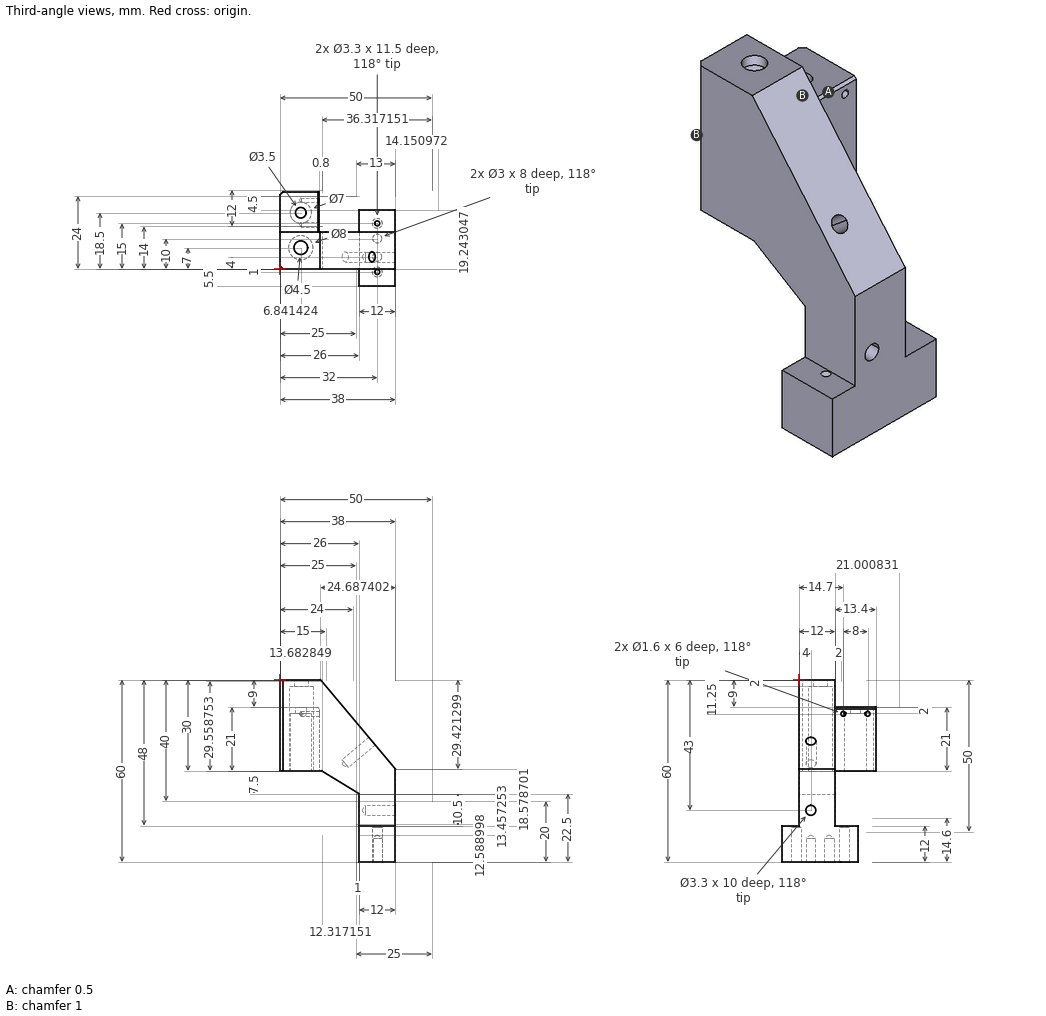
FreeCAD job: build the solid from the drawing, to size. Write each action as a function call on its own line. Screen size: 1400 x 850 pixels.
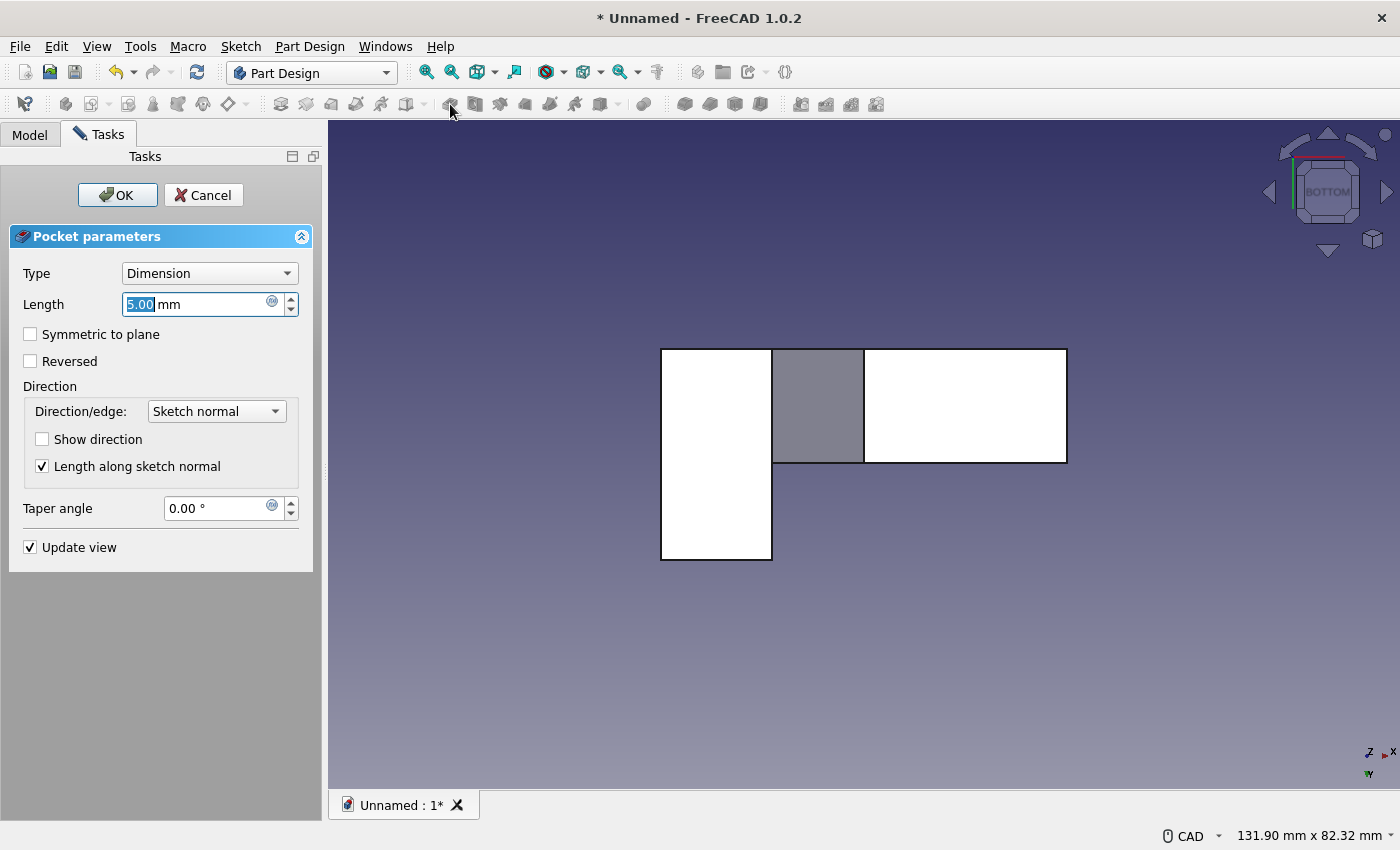
text(50)
key(Tab)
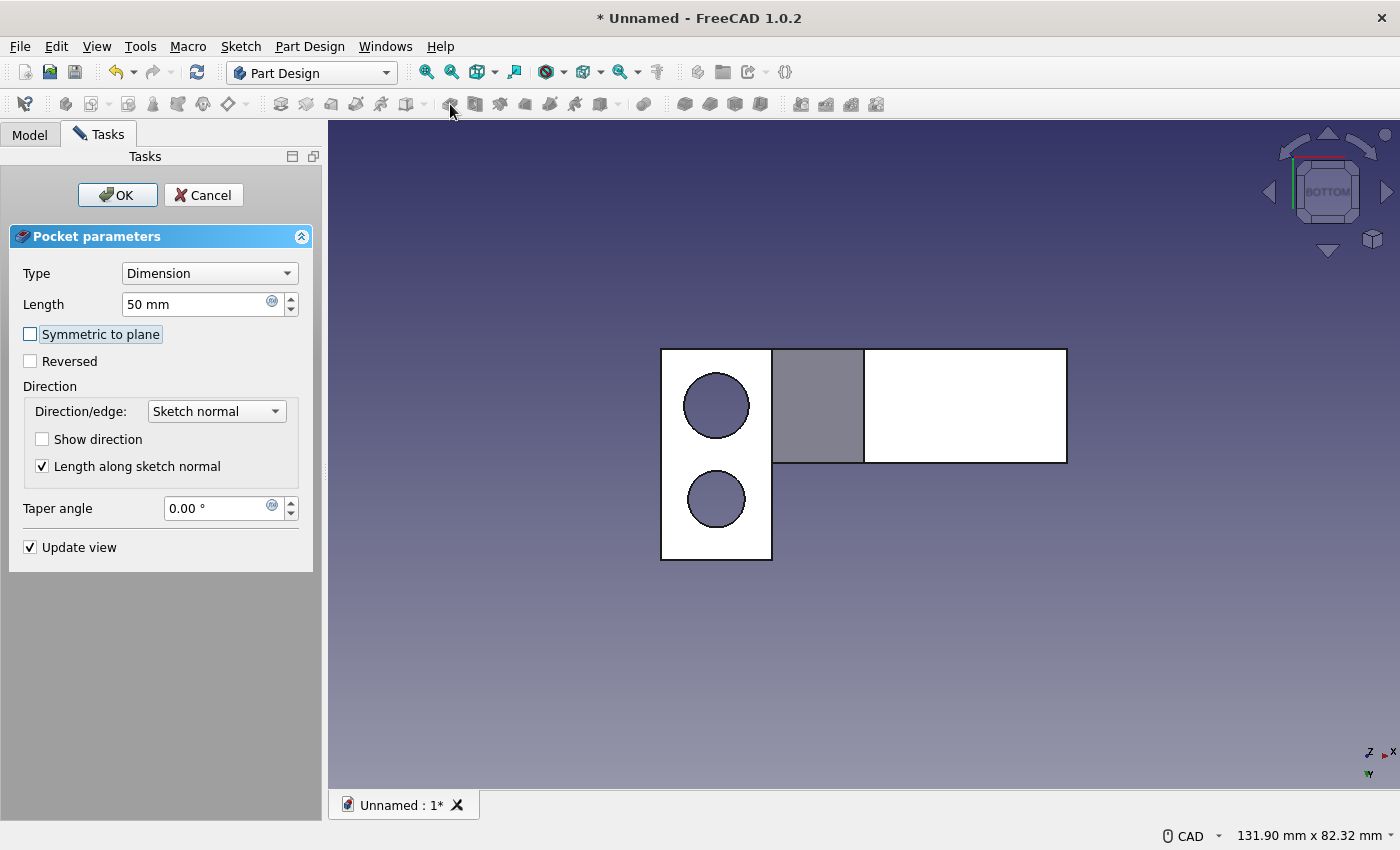
click(118, 195)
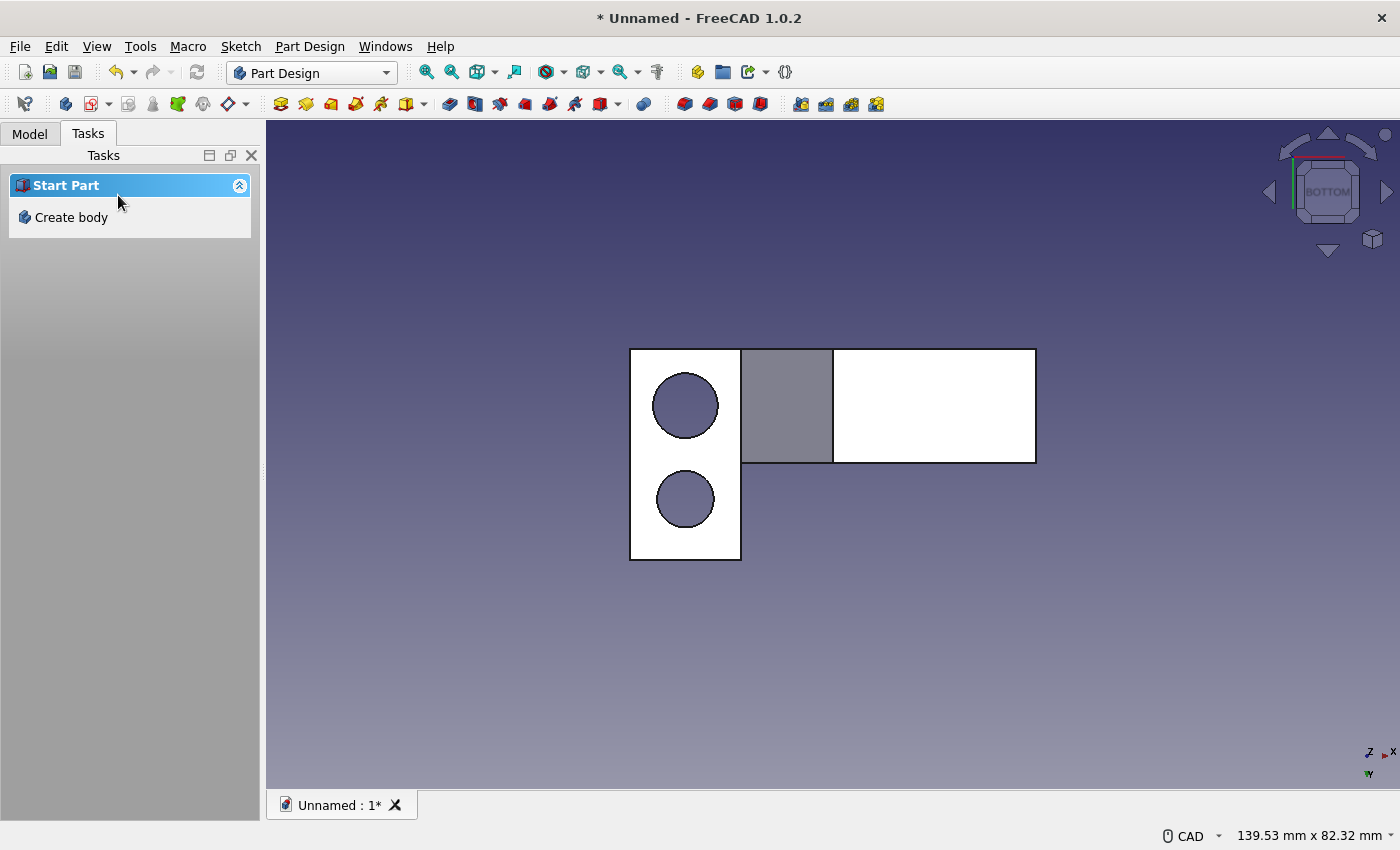
key(v)
key(f)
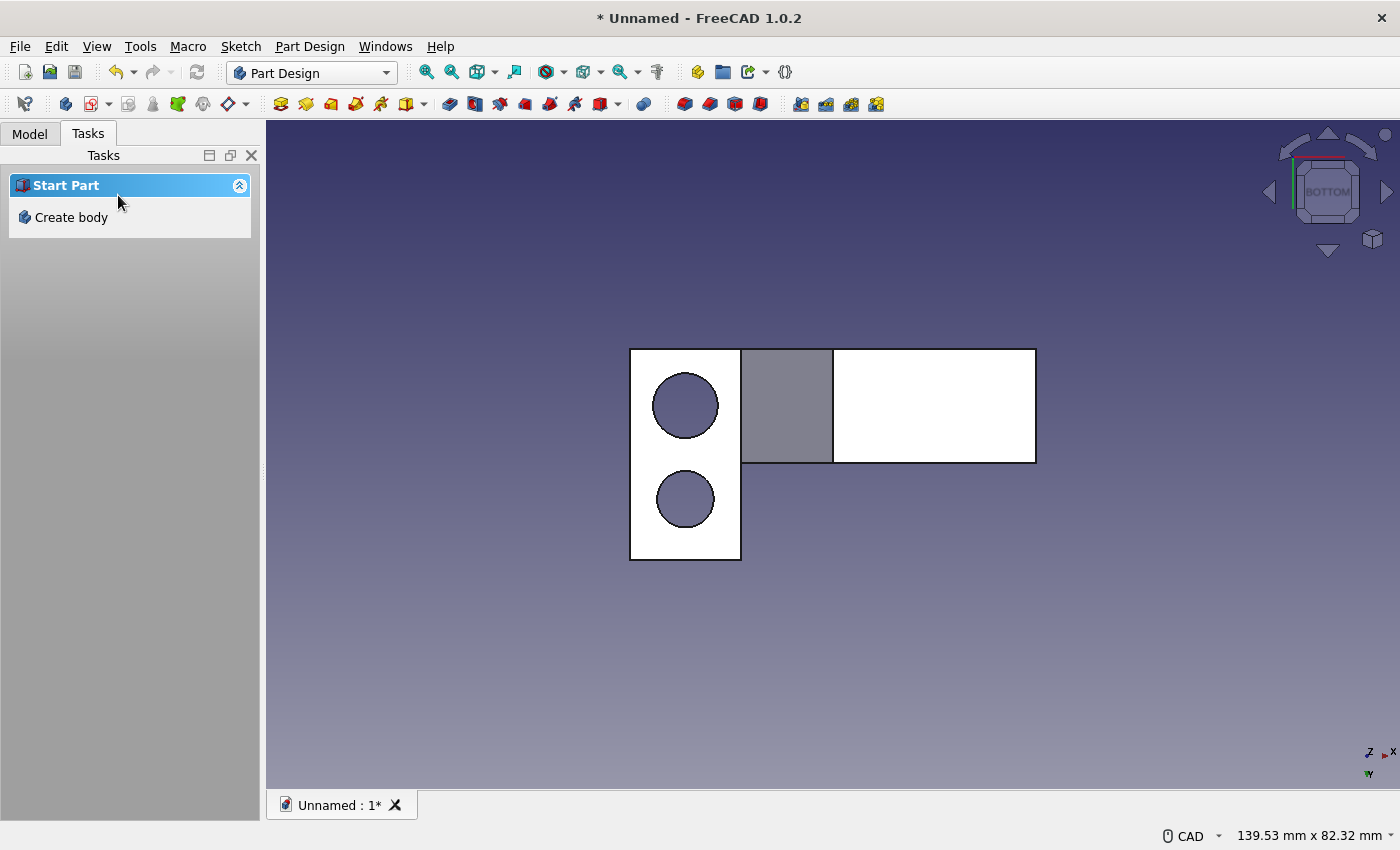
click(90, 104)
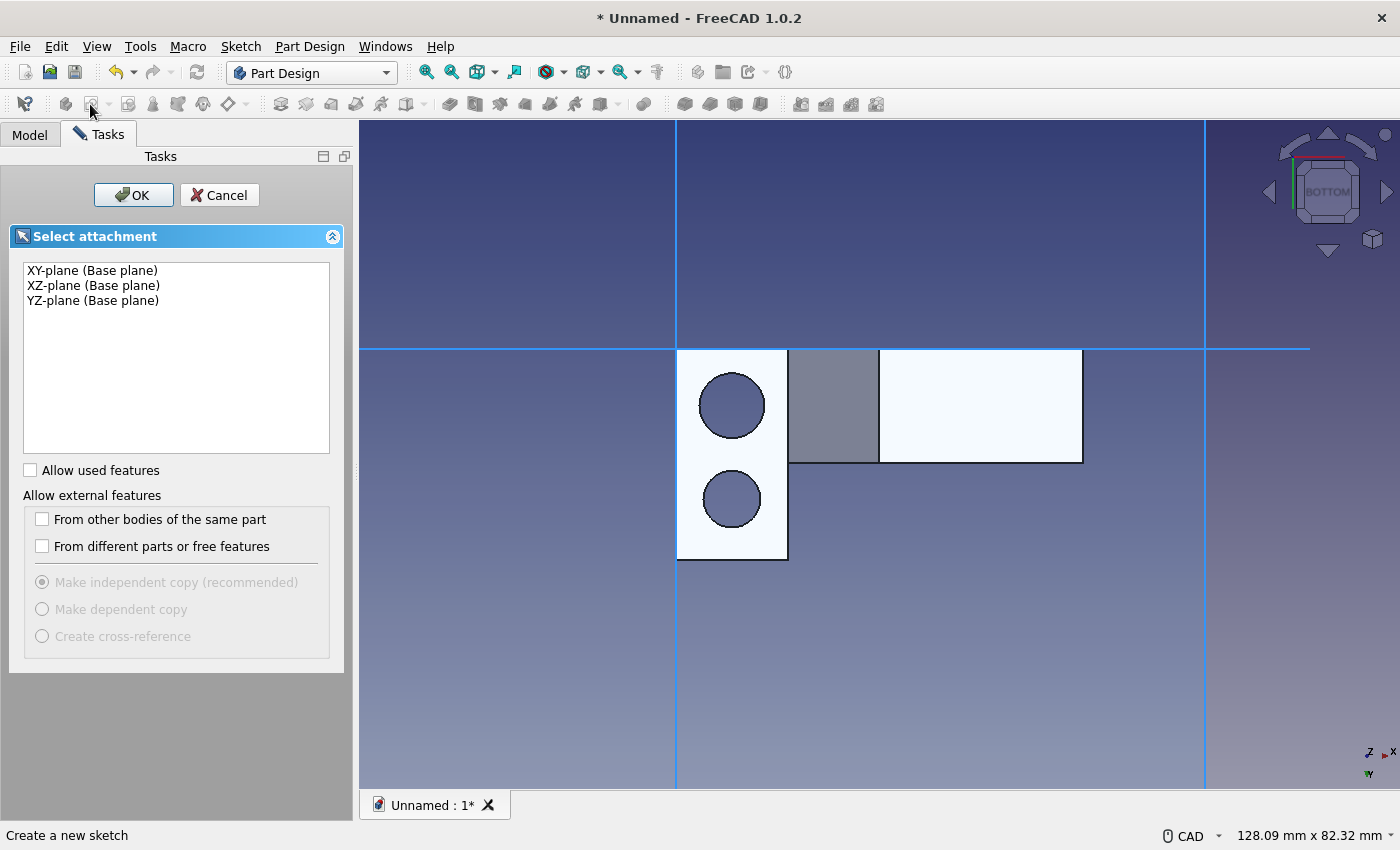
click(84, 270)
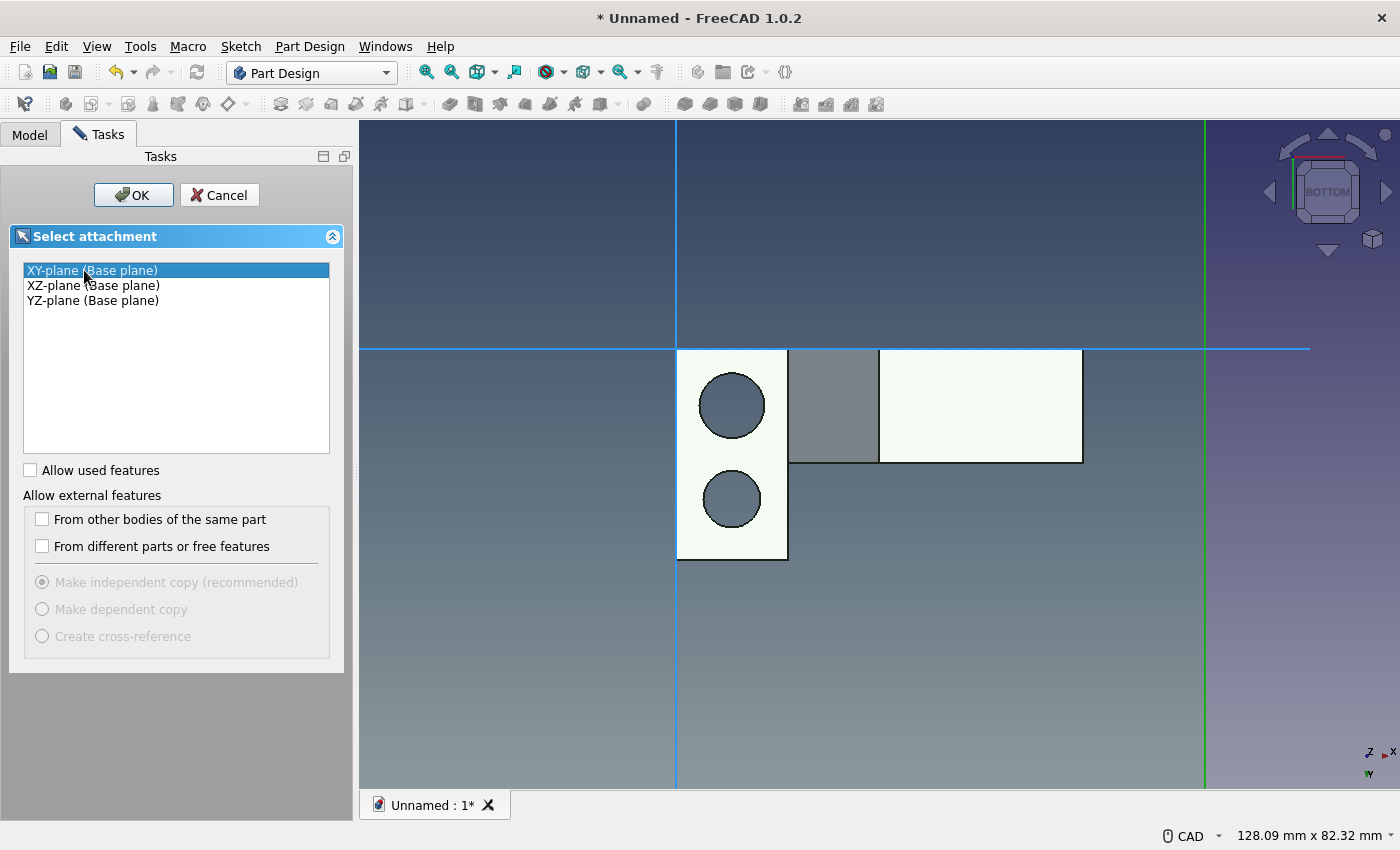
click(134, 195)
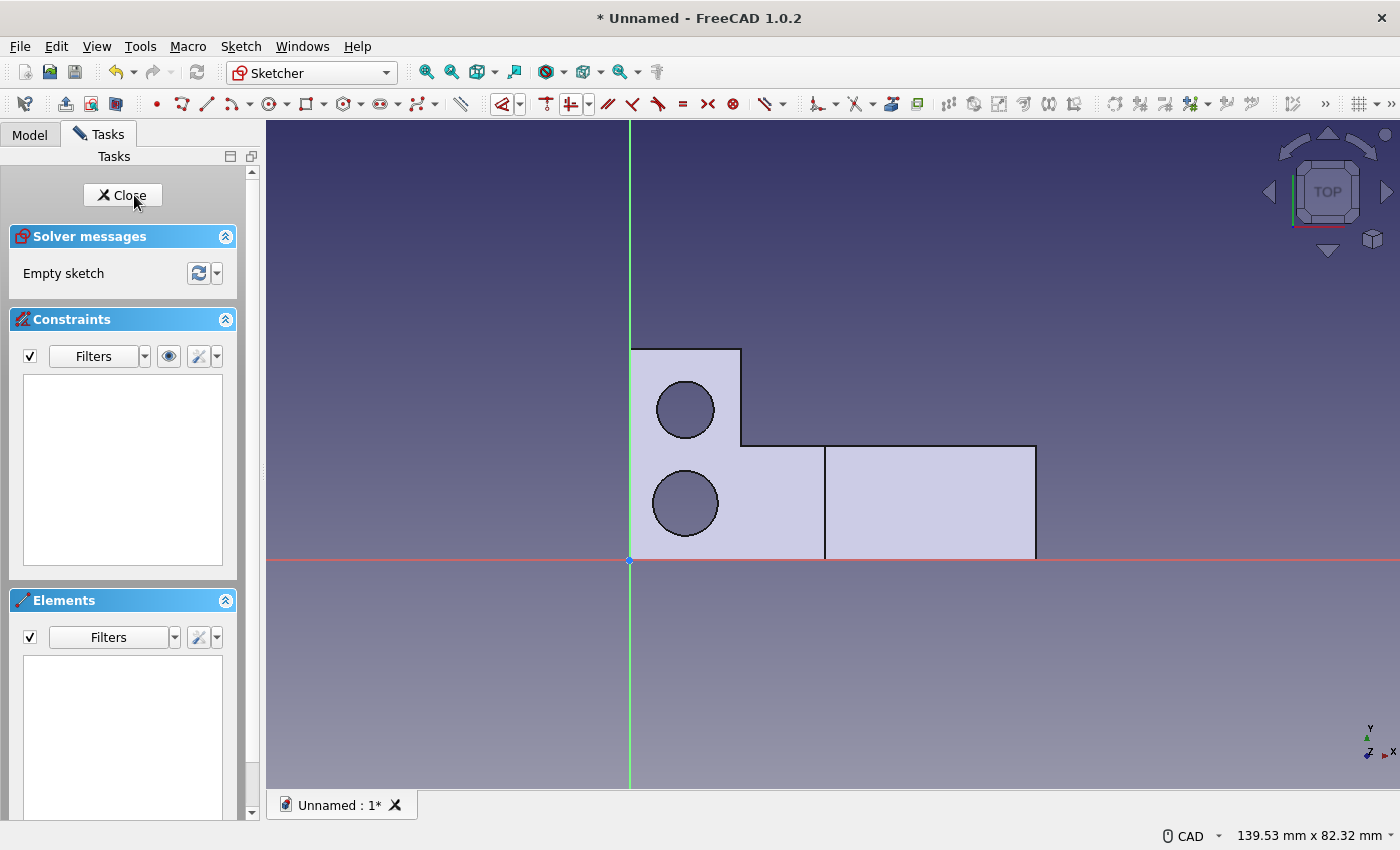
scroll(651, 531, up, 8)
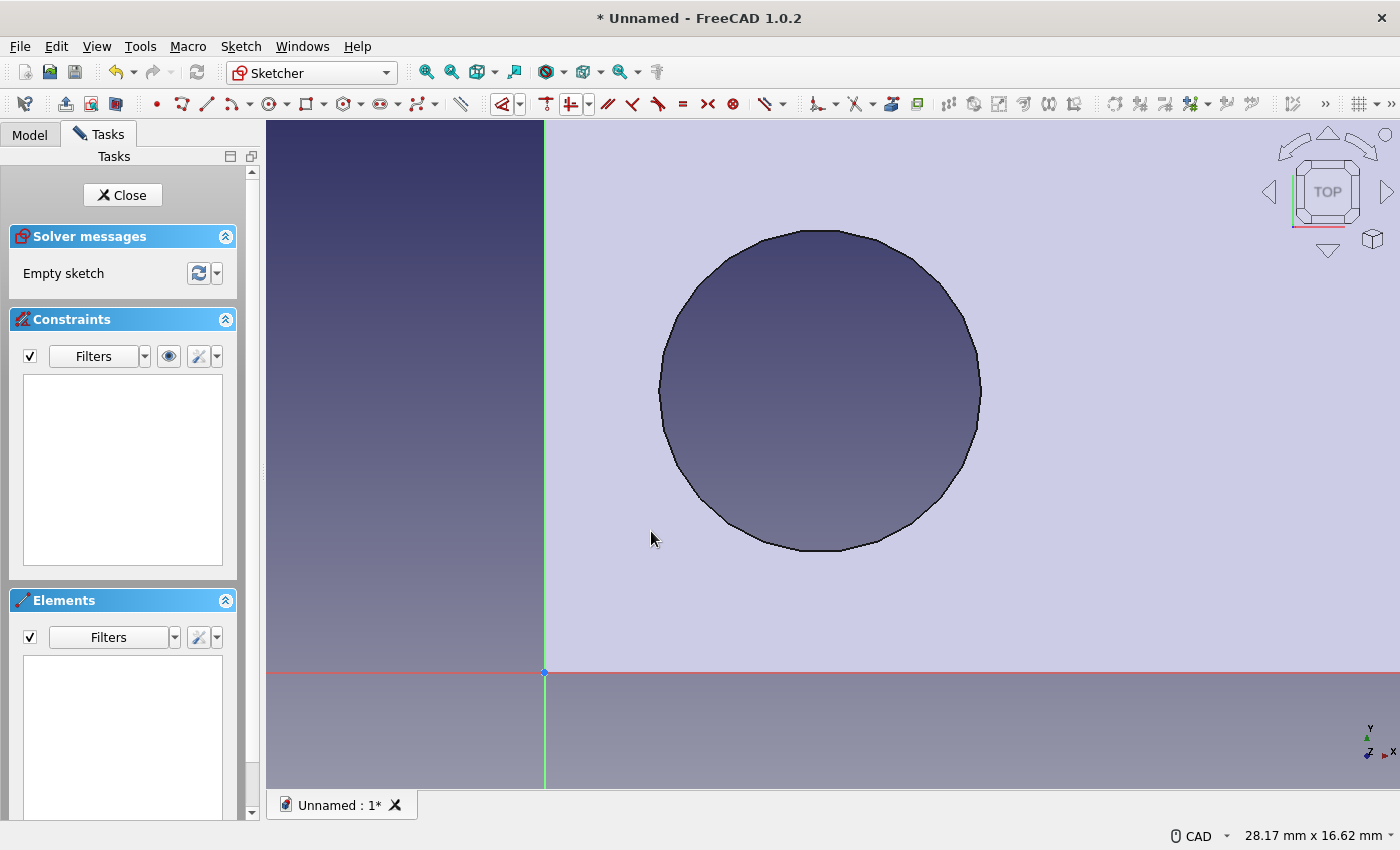
click(268, 104)